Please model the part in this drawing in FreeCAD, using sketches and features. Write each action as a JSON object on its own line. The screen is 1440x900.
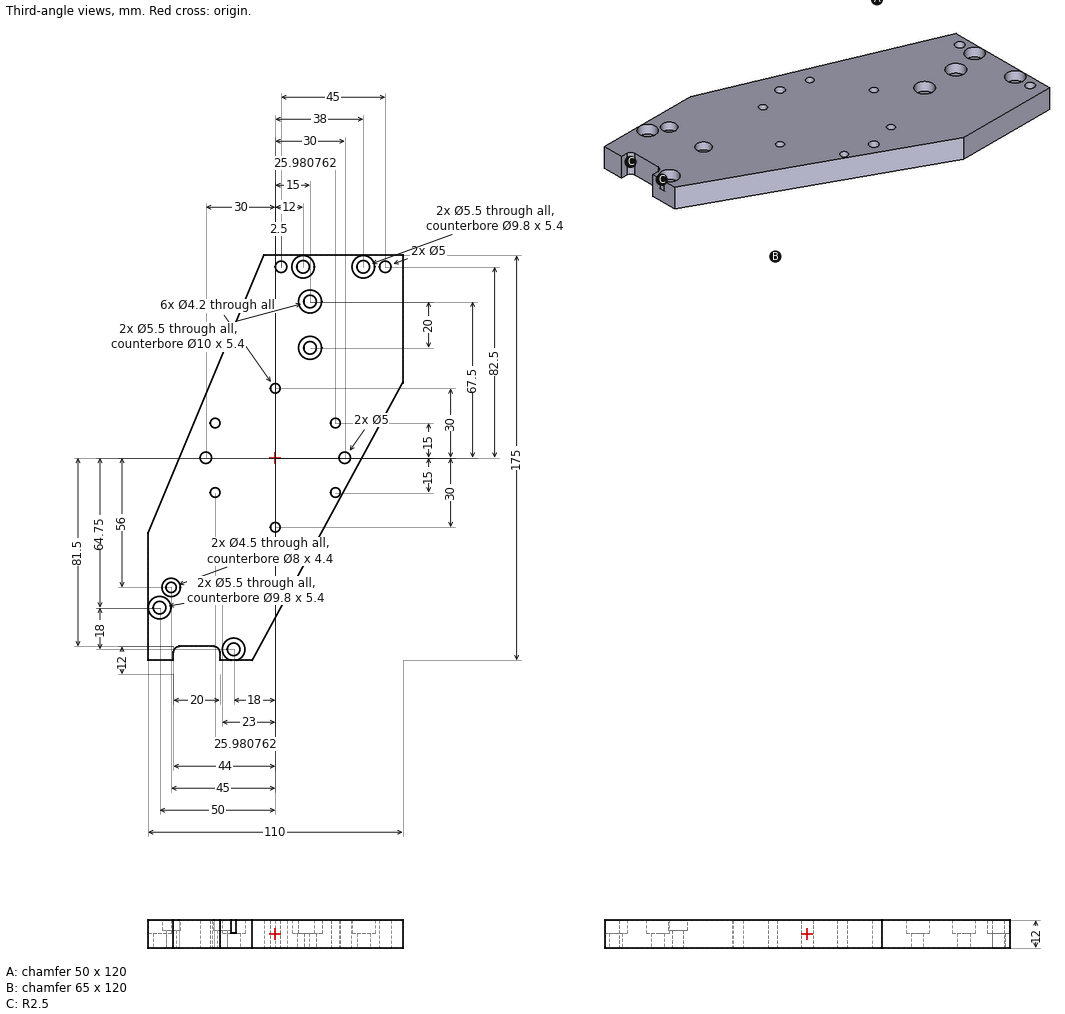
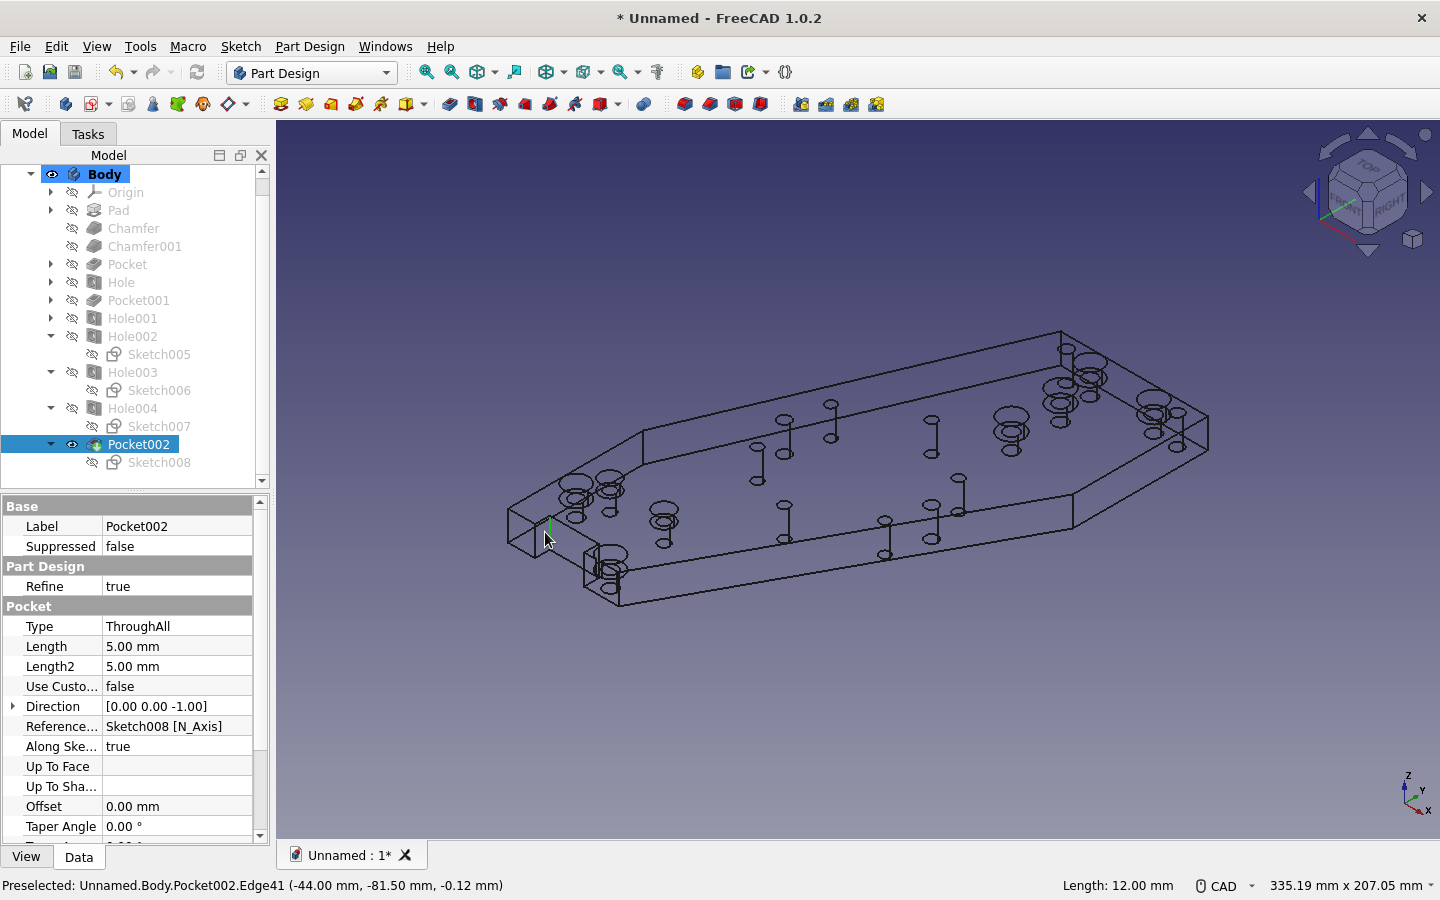
{"action": "scroll", "coordinate": [599, 560], "scroll_direction": "up", "scroll_amount": 6}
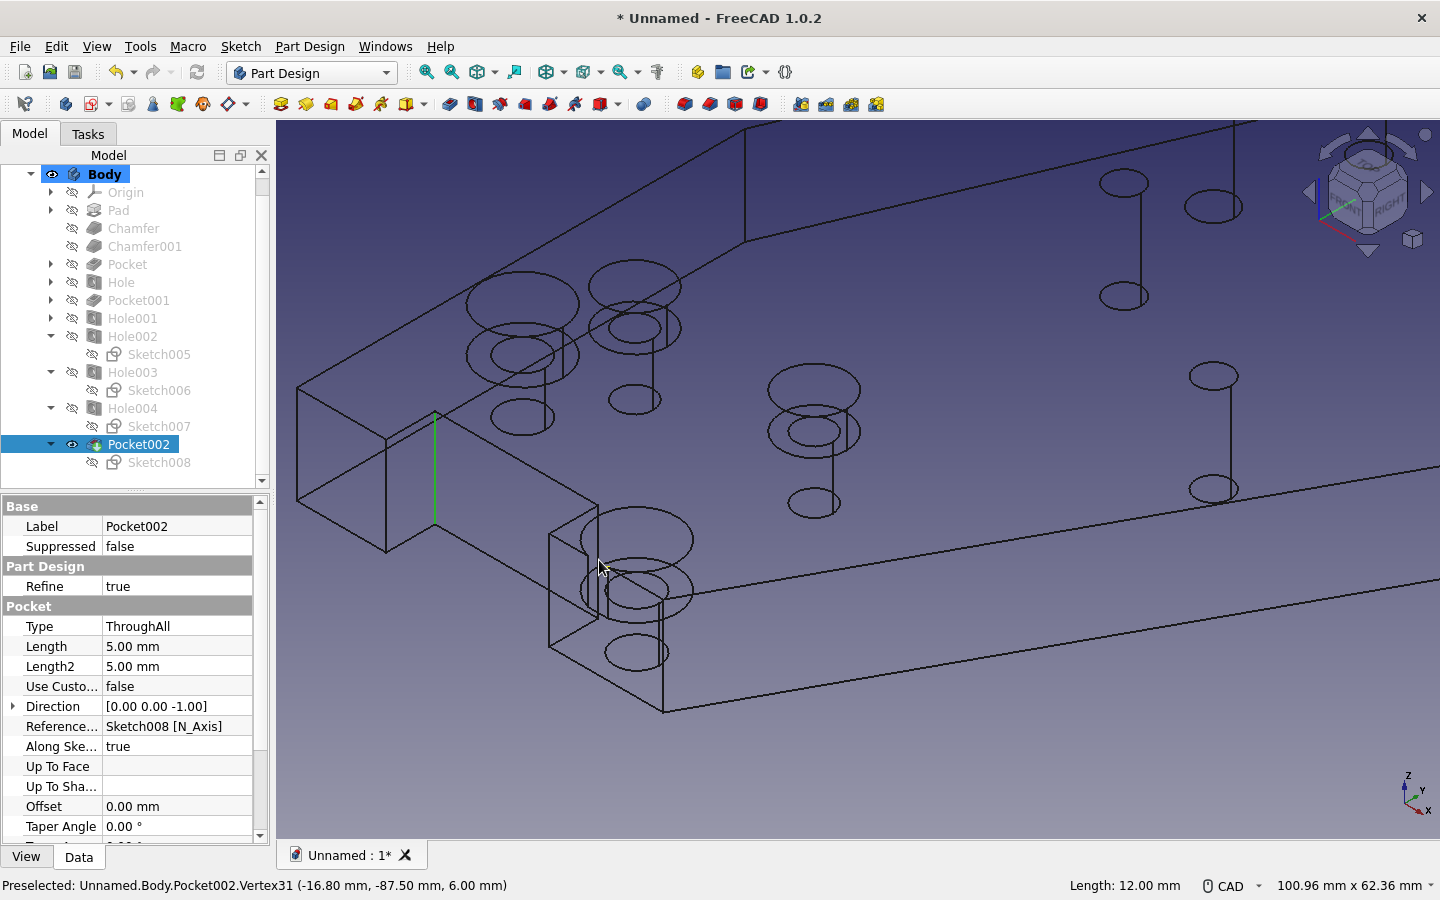
{"action": "left_click", "coordinate": [598, 550], "text": "ctrl"}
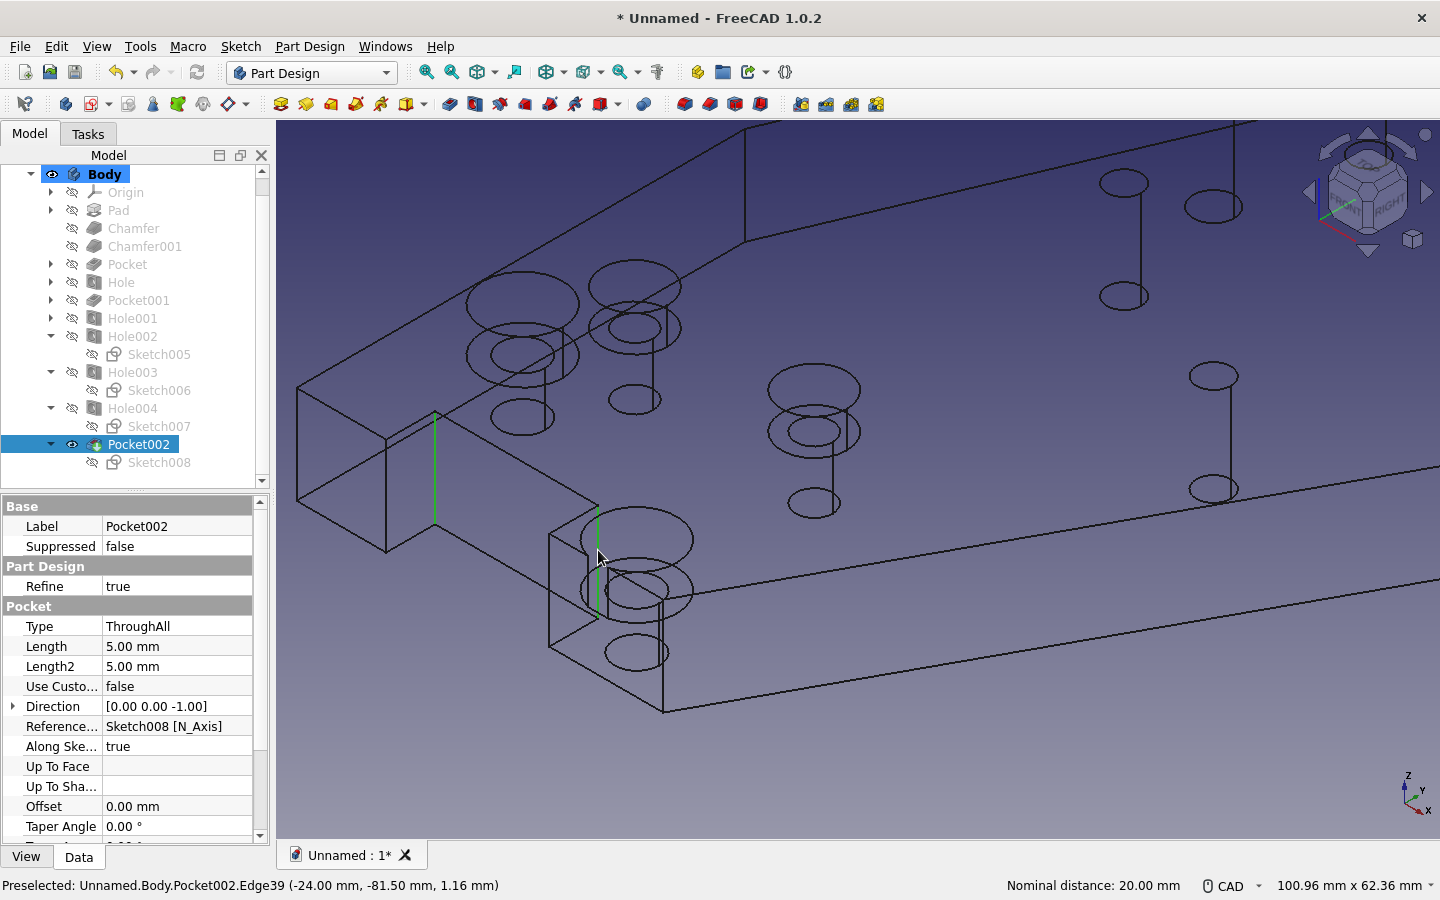
{"action": "key", "text": "v 1"}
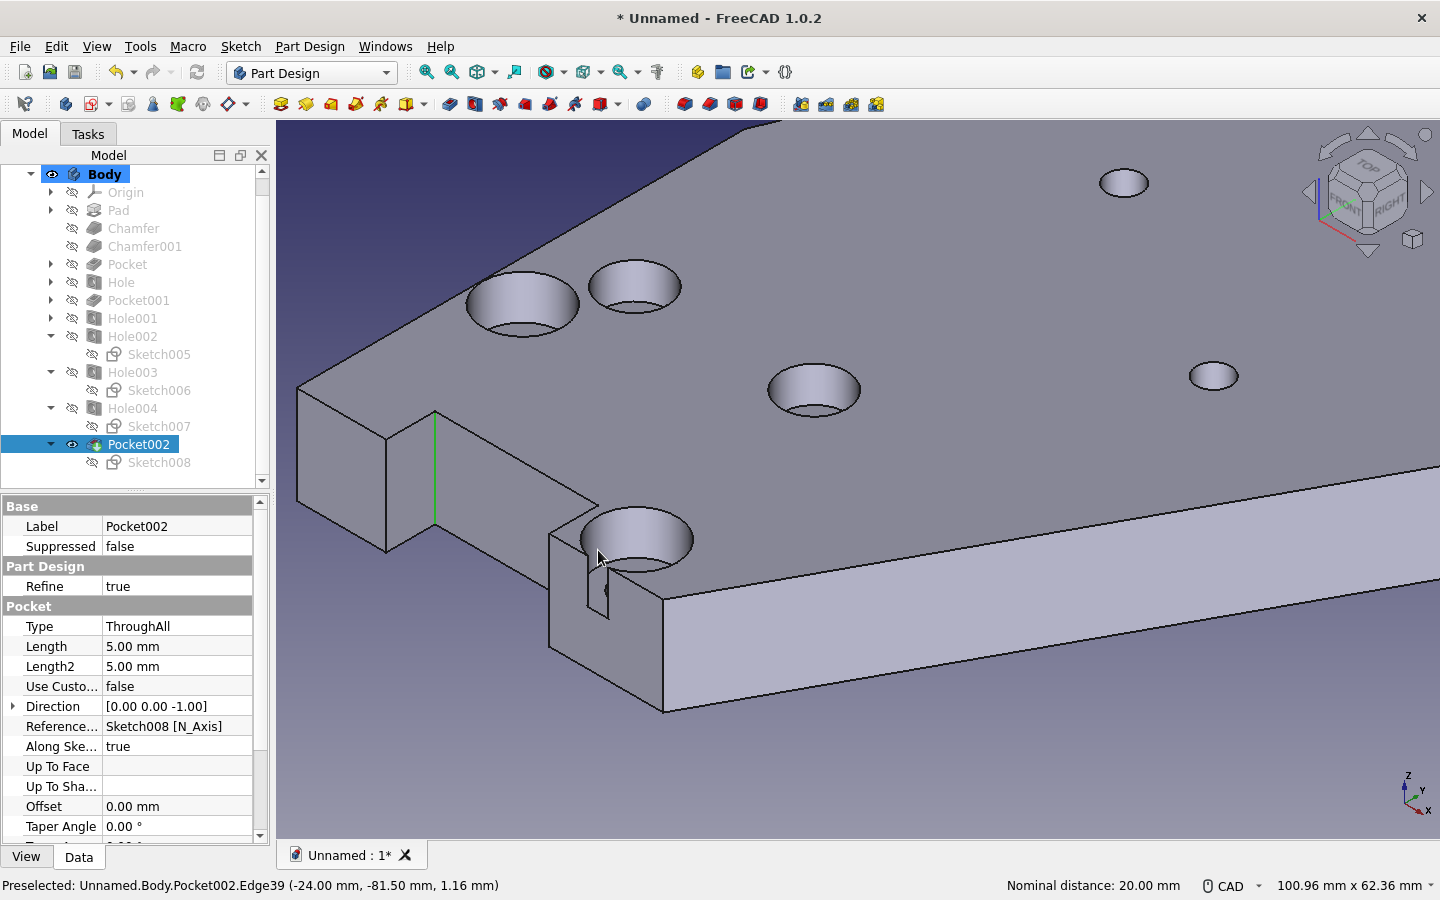
{"action": "left_click", "coordinate": [685, 104]}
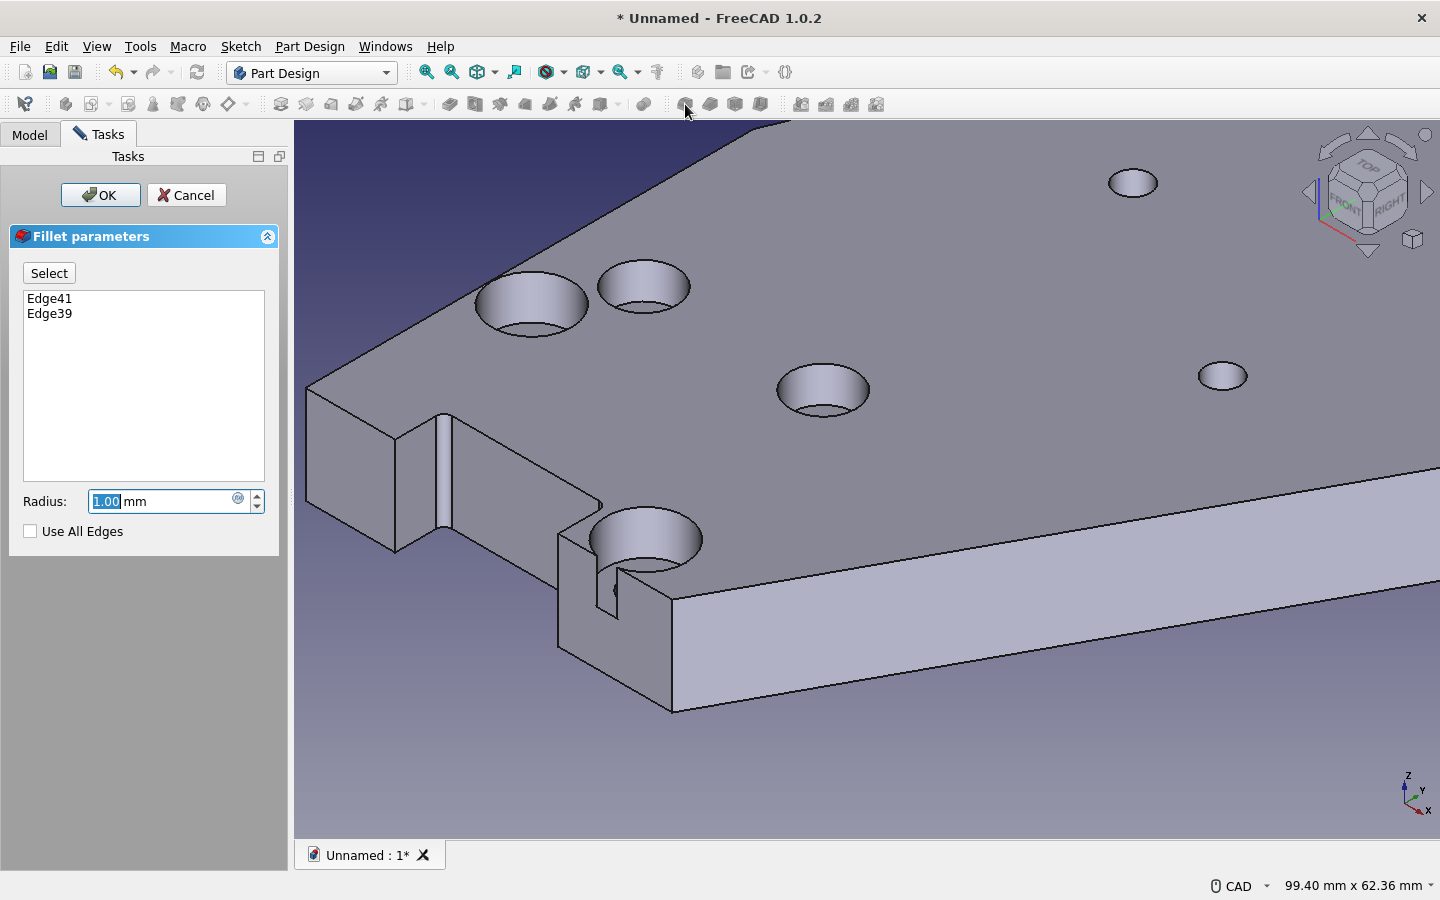
{"action": "type", "text": "2.5"}
{"action": "key", "text": "Tab"}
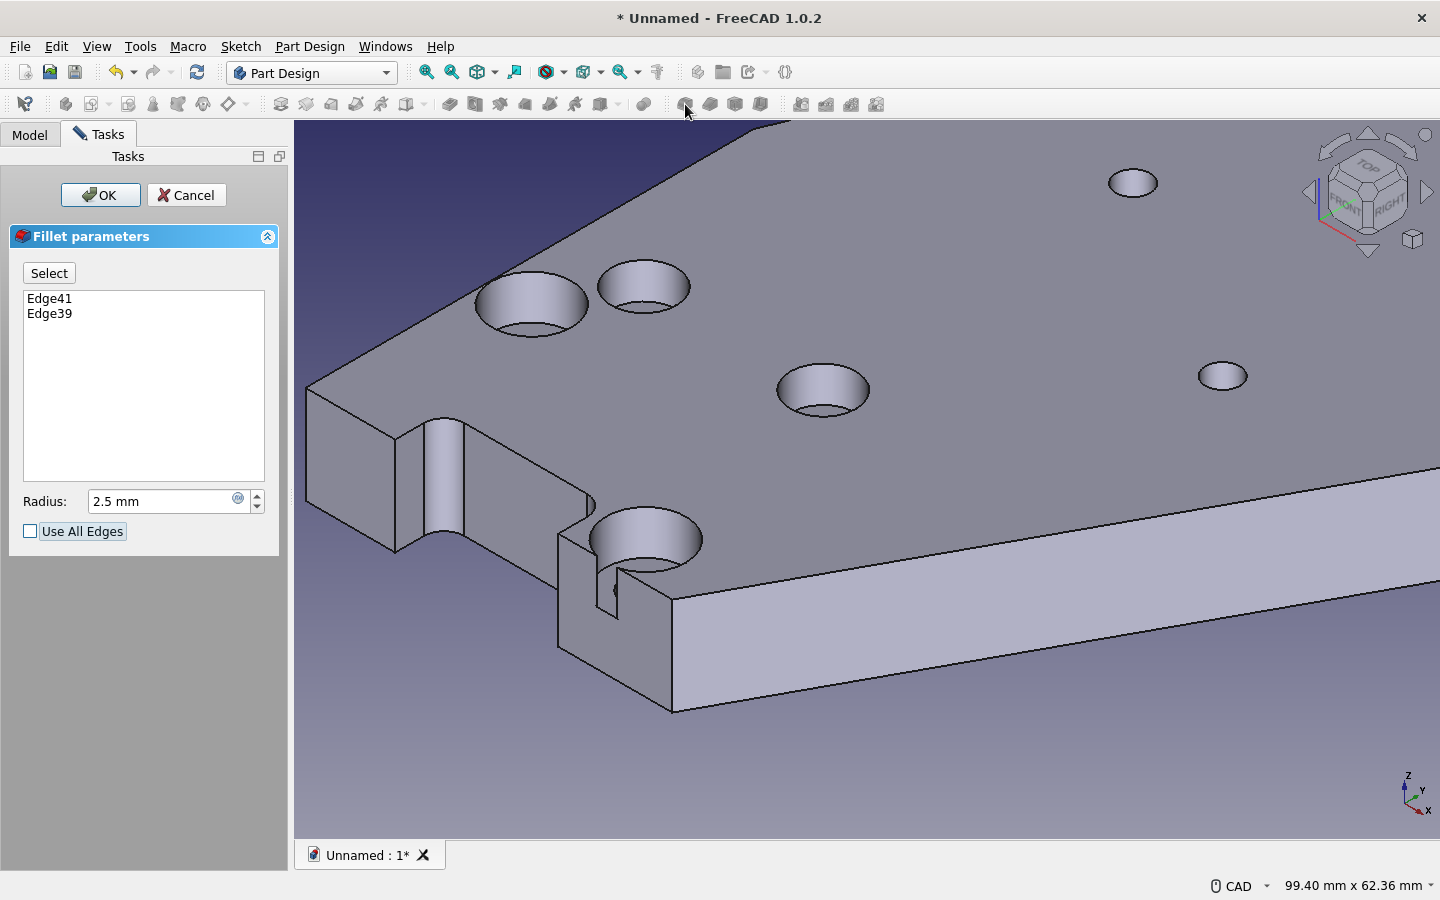
{"action": "left_click", "coordinate": [101, 195]}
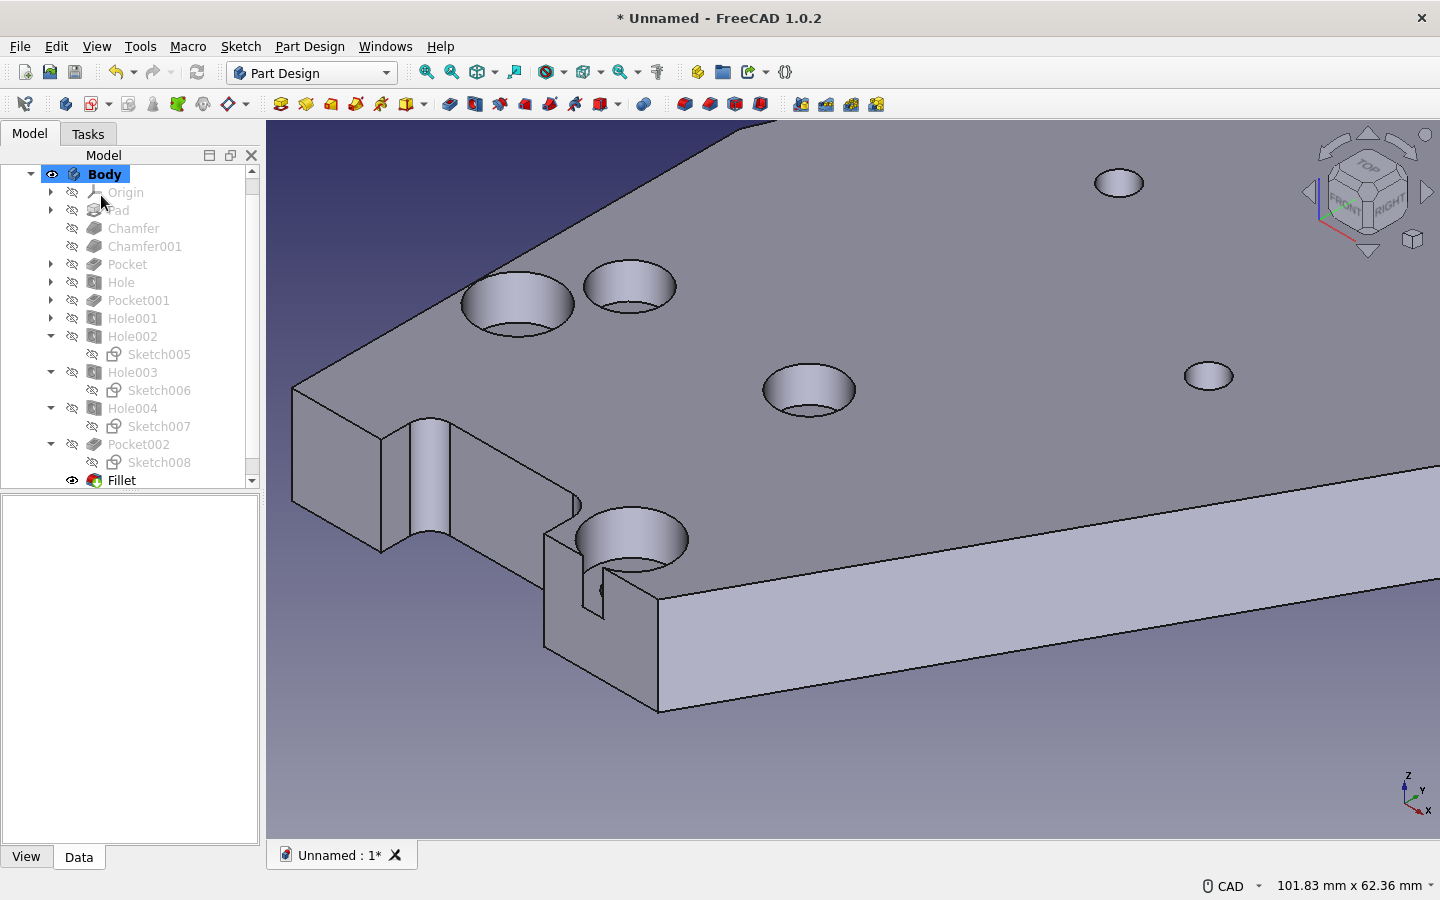
{"action": "key", "text": "v f"}